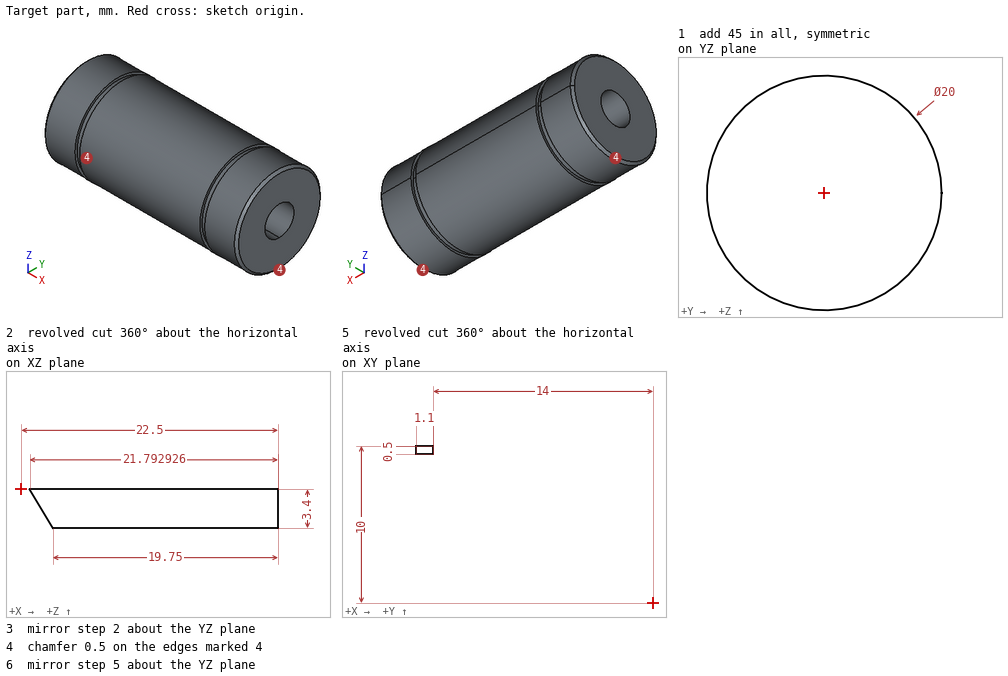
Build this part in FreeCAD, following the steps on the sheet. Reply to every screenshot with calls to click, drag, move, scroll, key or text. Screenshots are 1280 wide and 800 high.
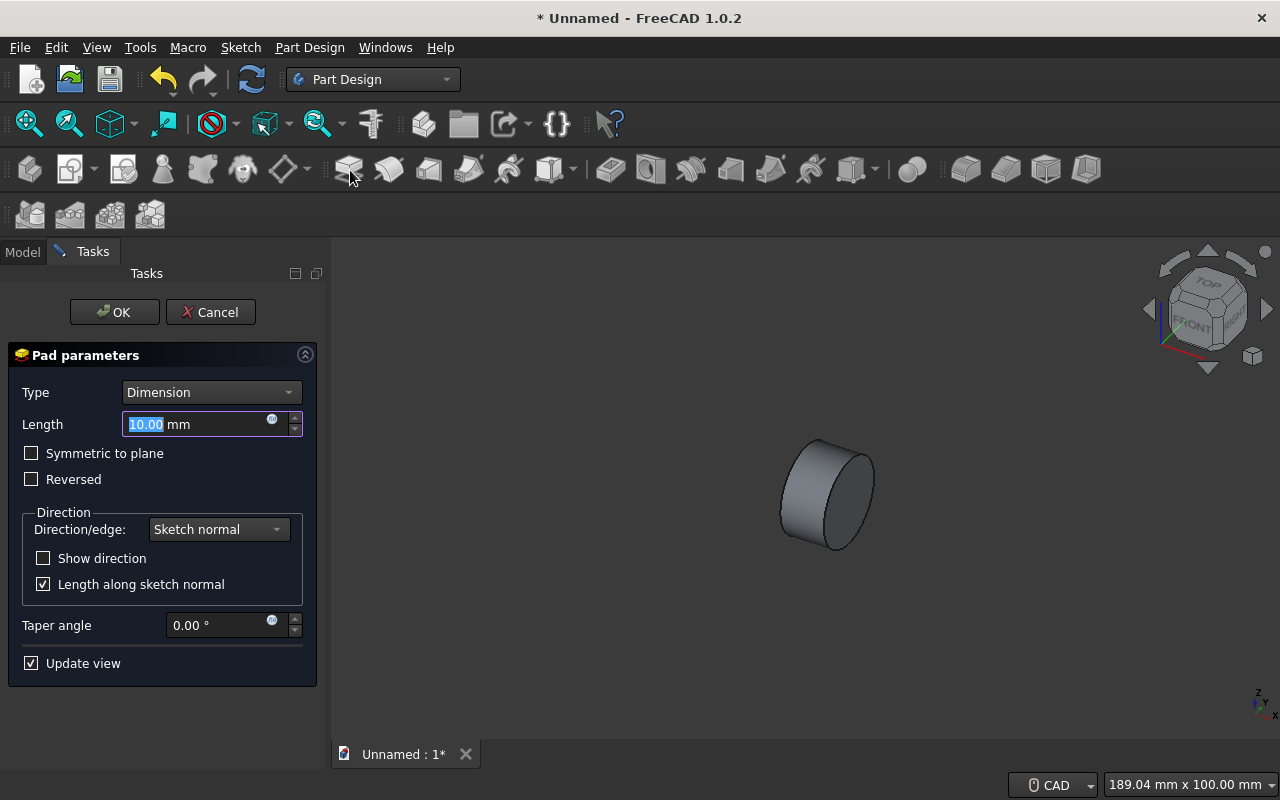
text(45)
key(Tab)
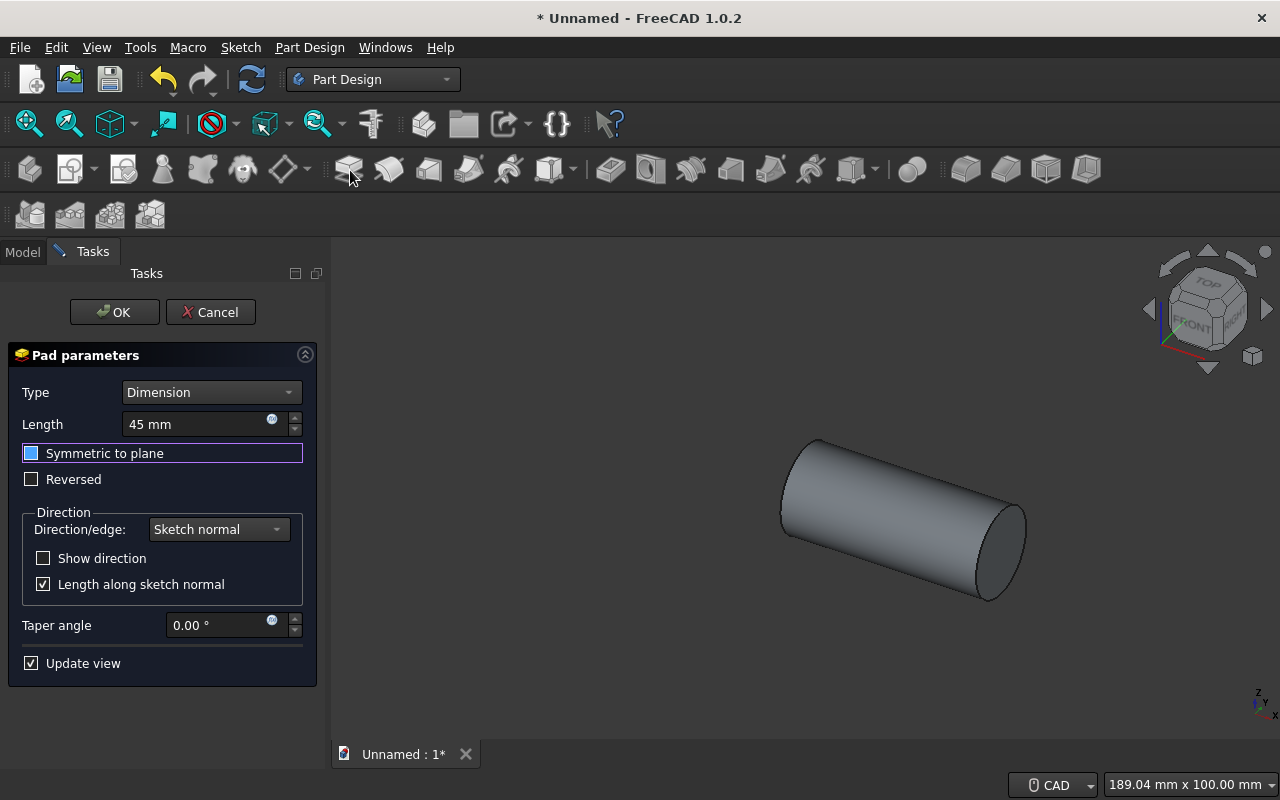
click(30, 453)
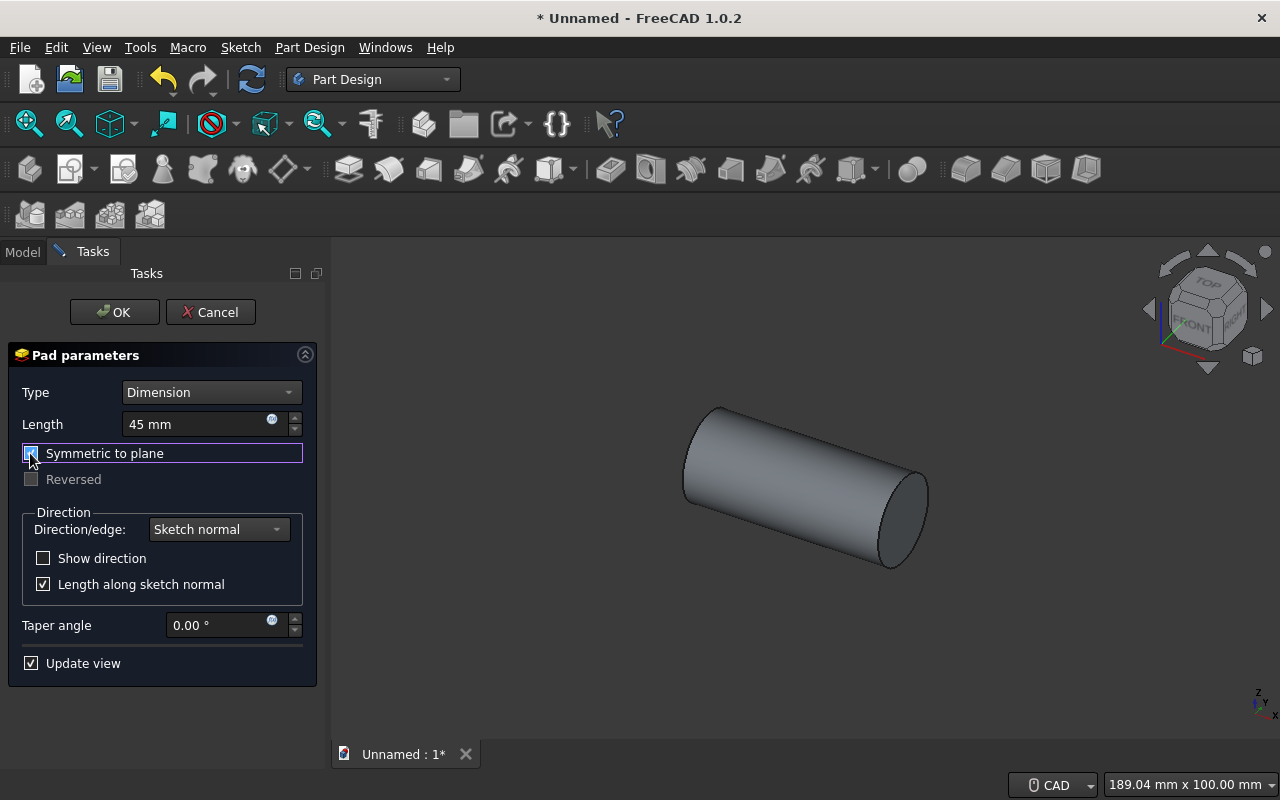
click(115, 312)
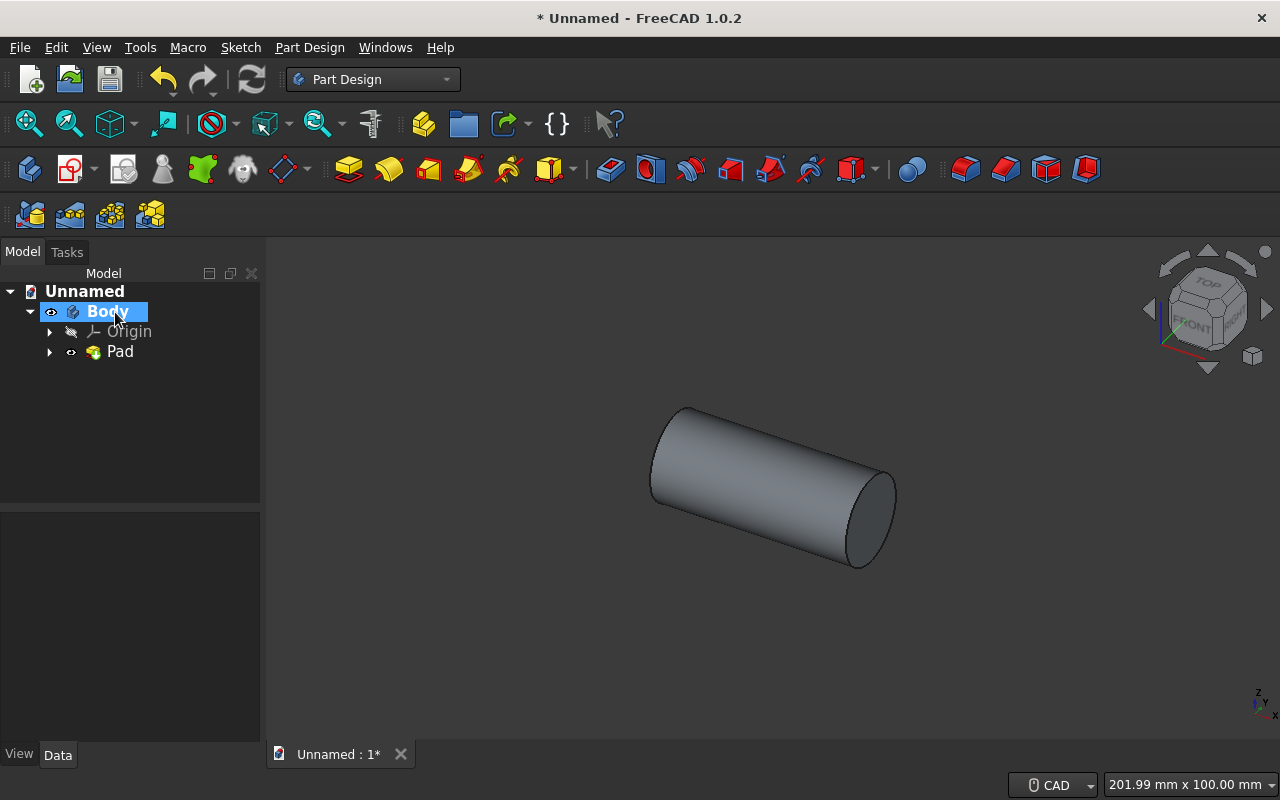
click(30, 124)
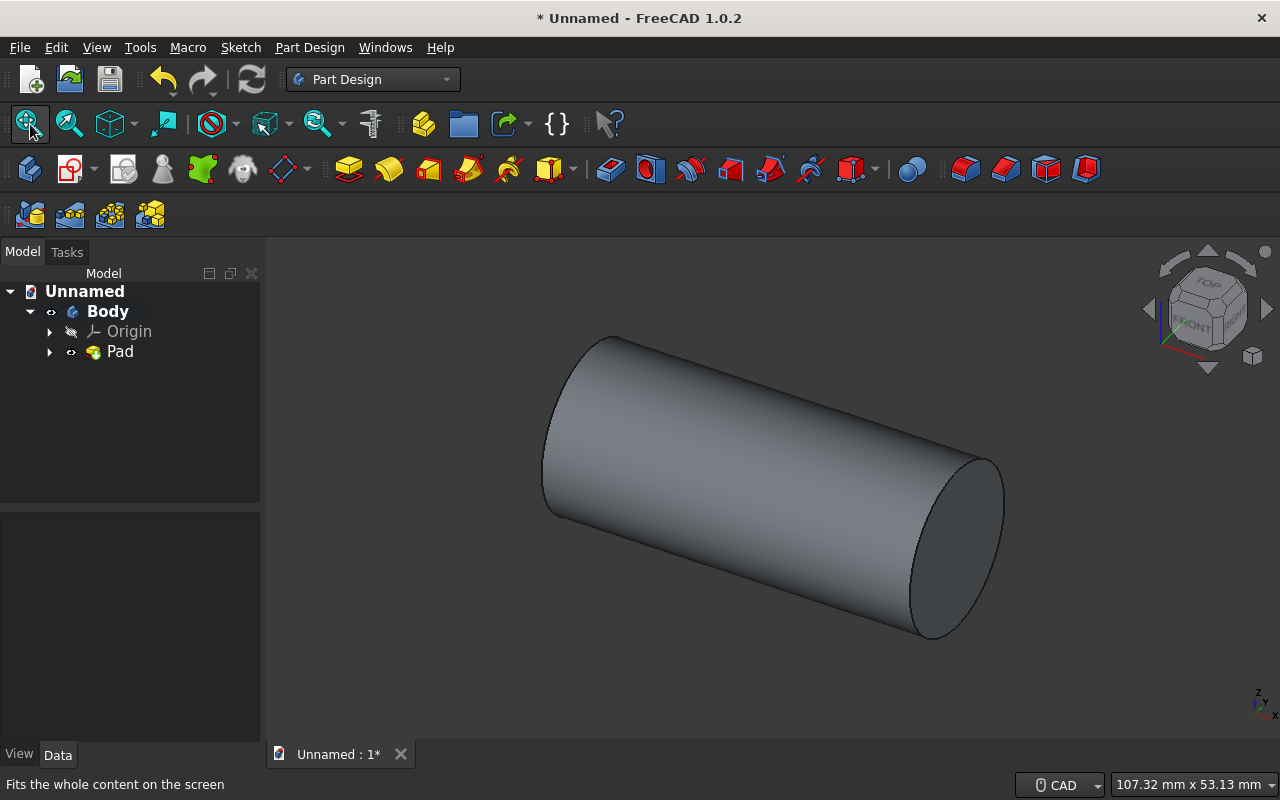
click(70, 170)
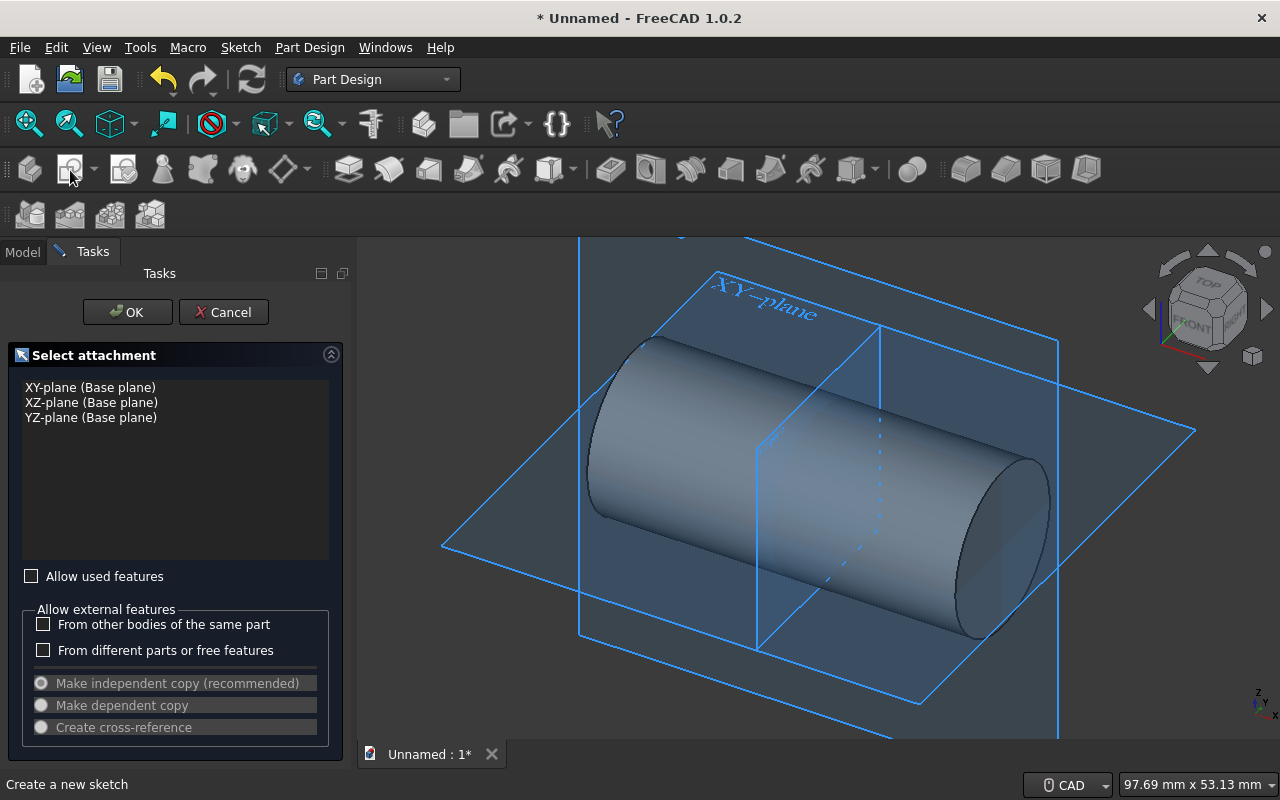
click(82, 402)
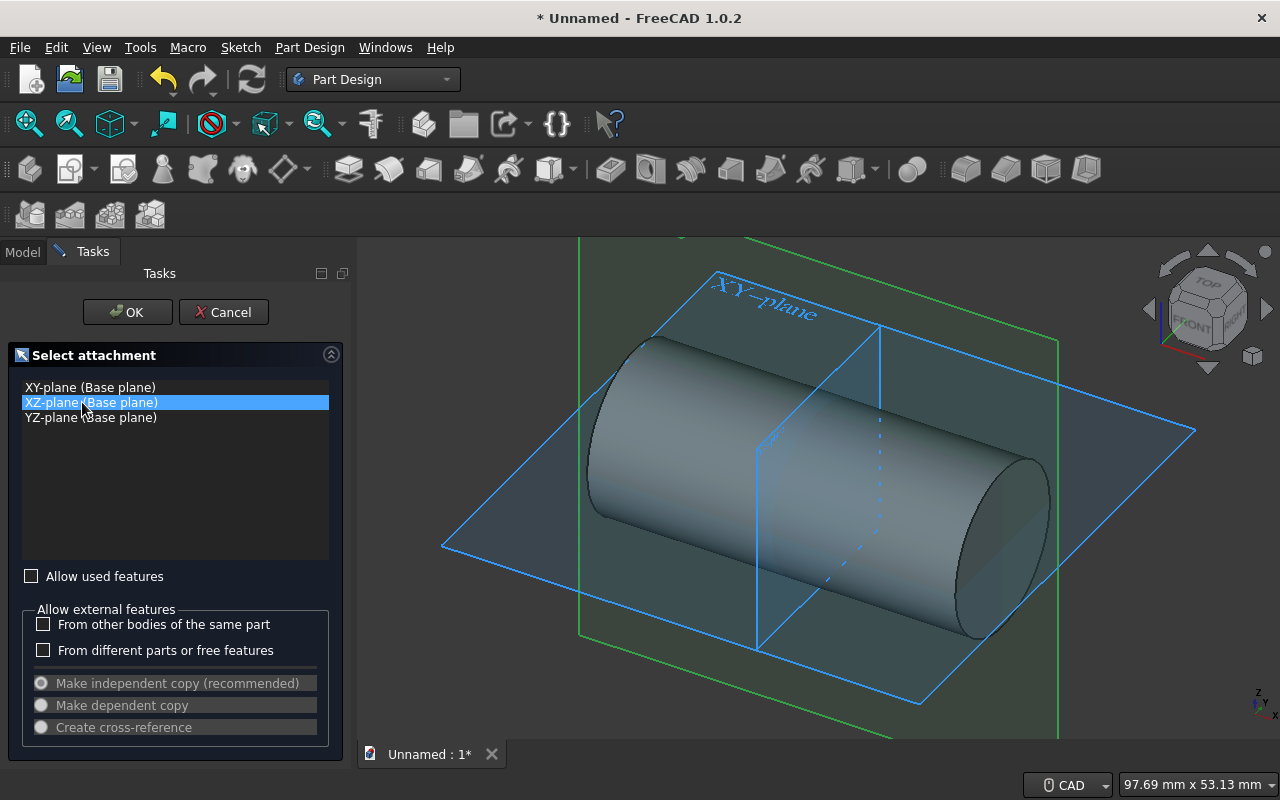
click(128, 312)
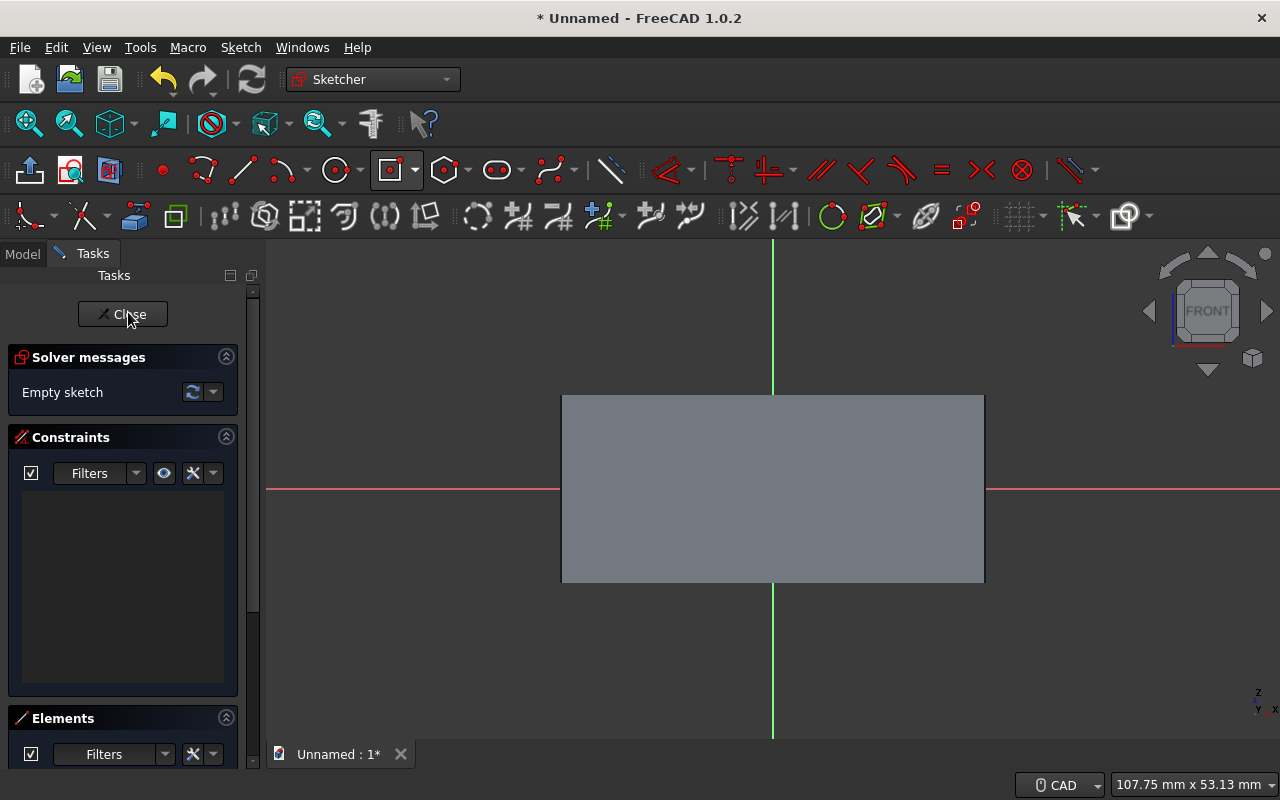
key(q)
key(s)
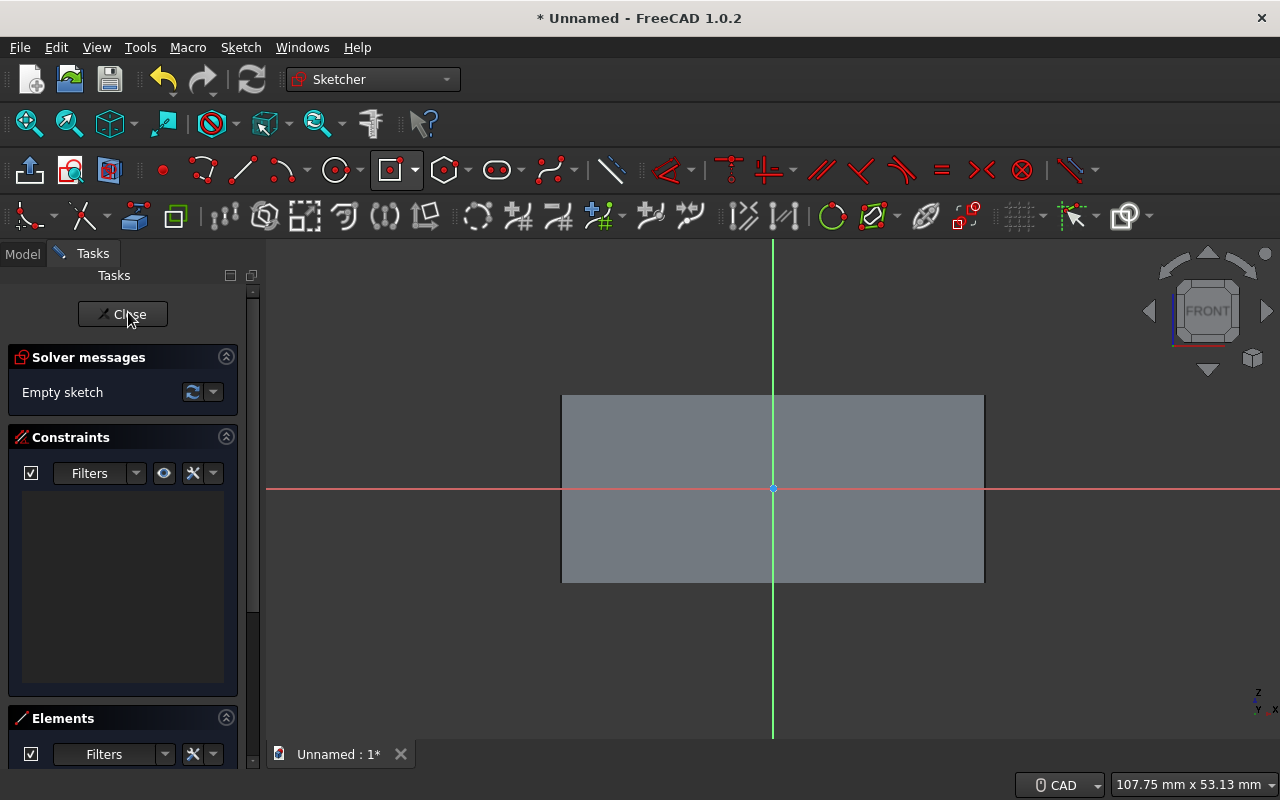
scroll(980, 514, up, 5)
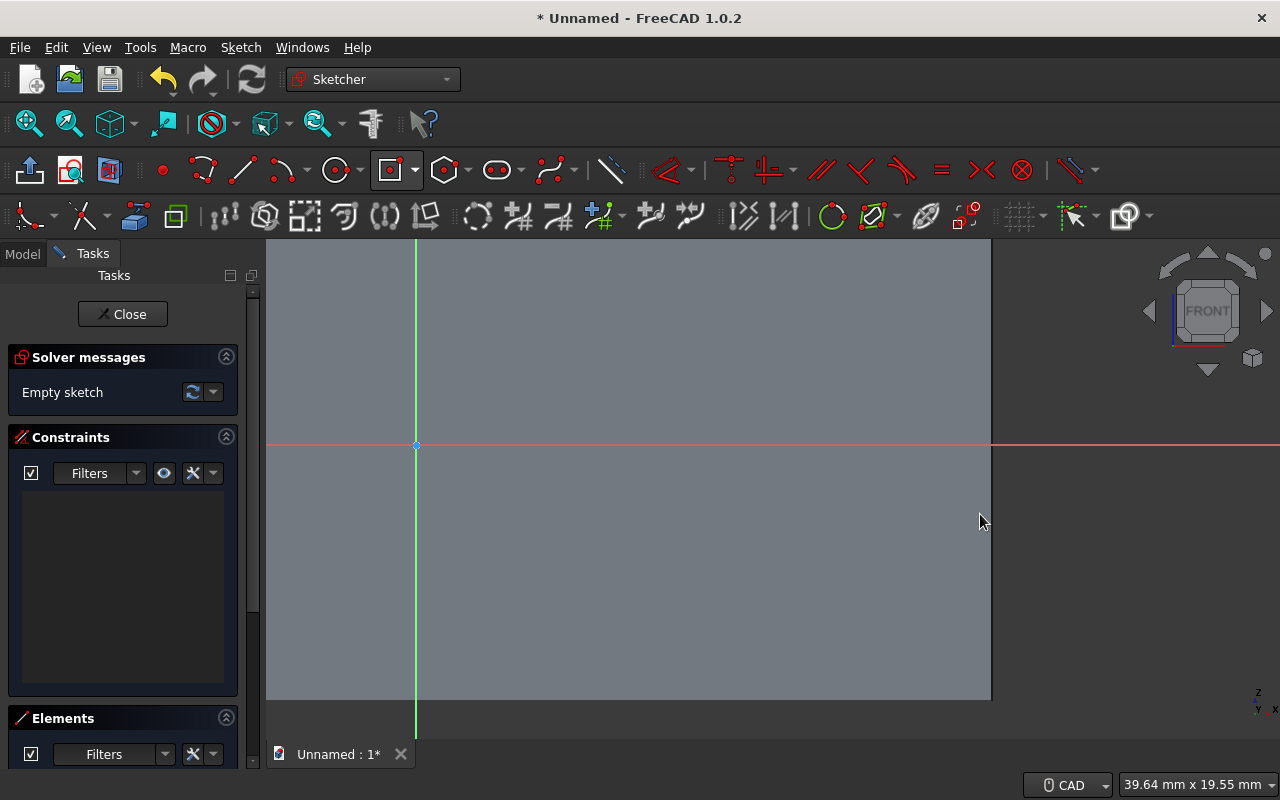
click(204, 170)